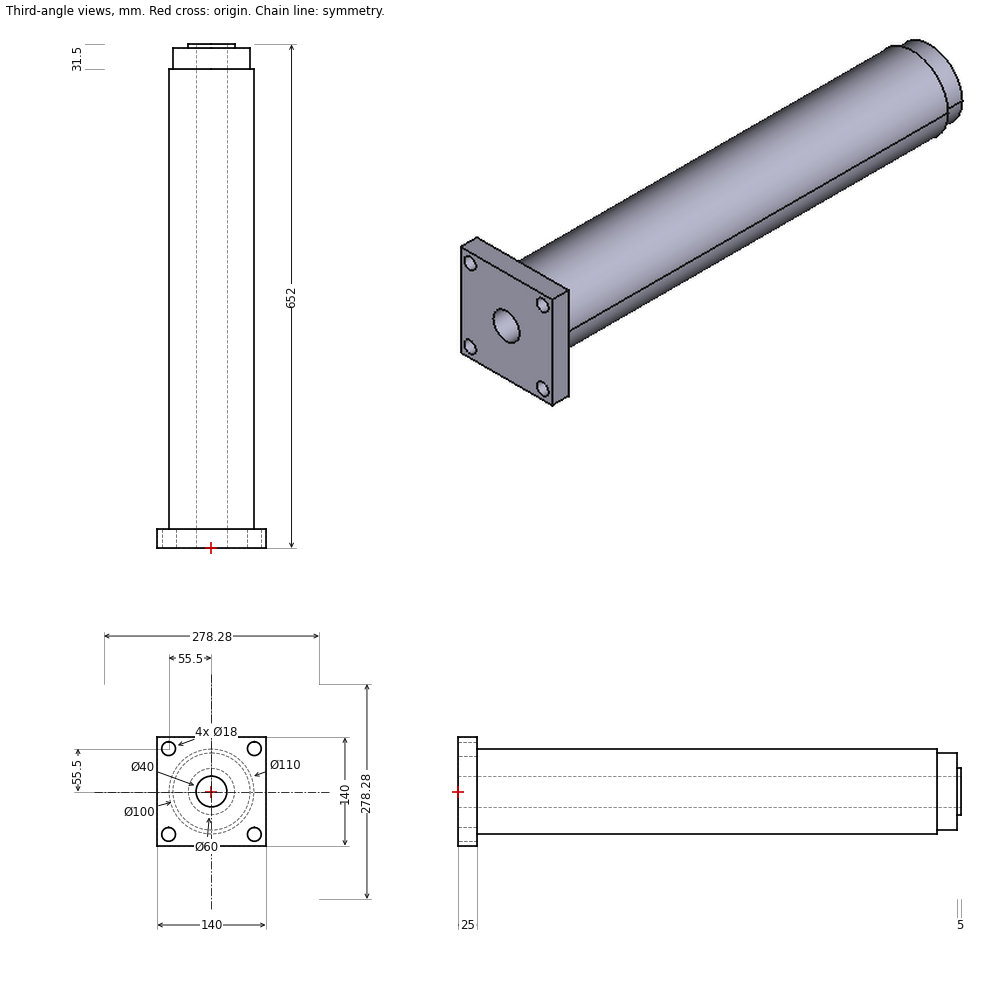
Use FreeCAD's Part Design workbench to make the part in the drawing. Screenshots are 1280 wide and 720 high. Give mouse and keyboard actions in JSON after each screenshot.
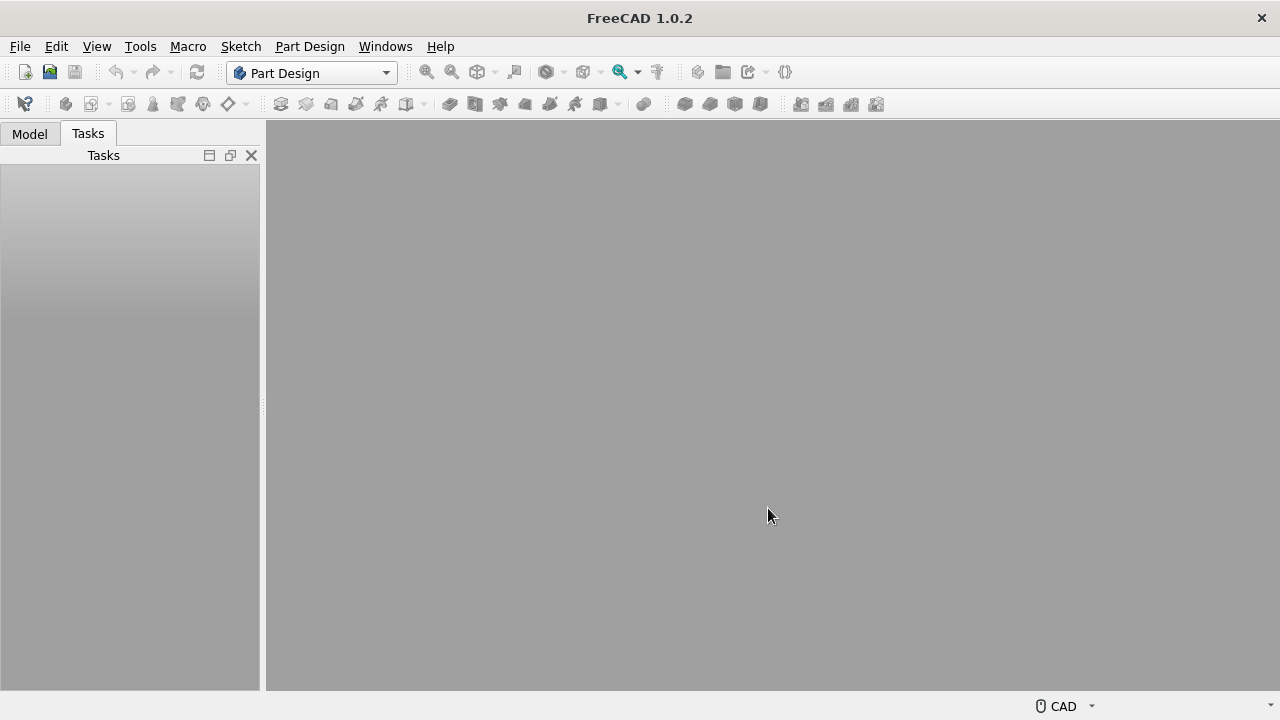
{"action": "left_click", "coordinate": [25, 72]}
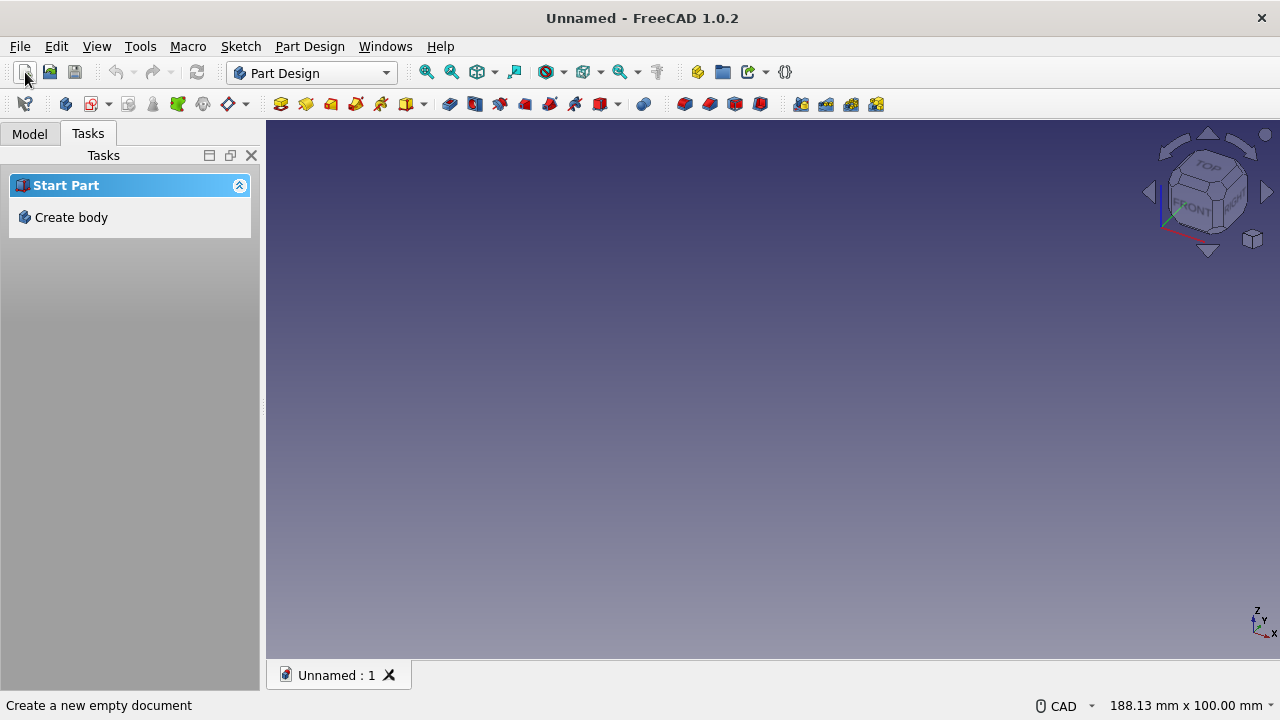
{"action": "left_click", "coordinate": [90, 104]}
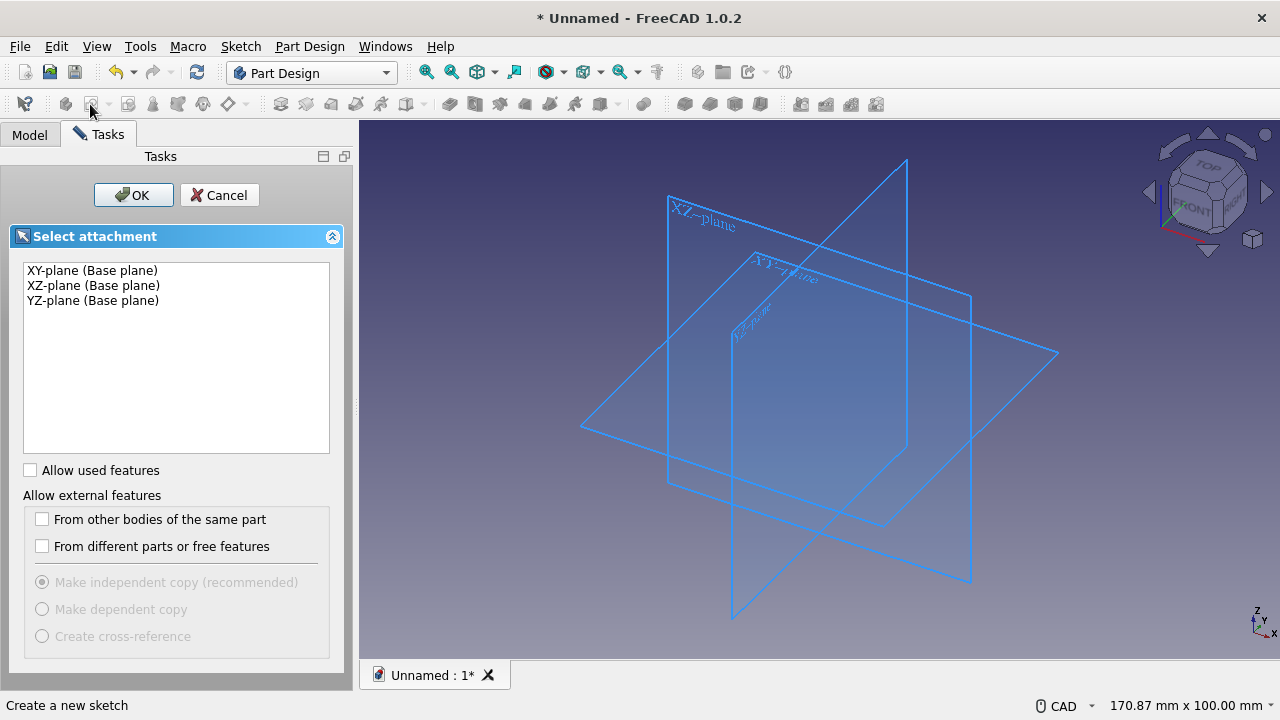
{"action": "left_click", "coordinate": [84, 286]}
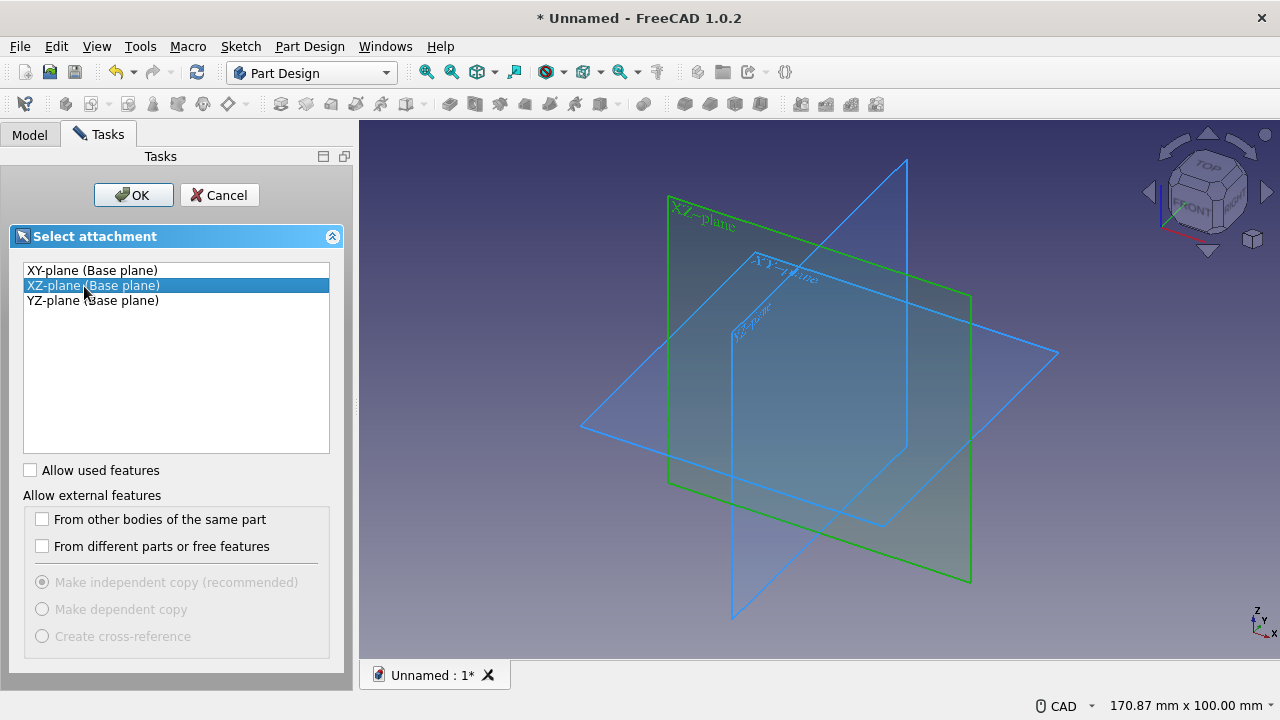
{"action": "left_click", "coordinate": [134, 195]}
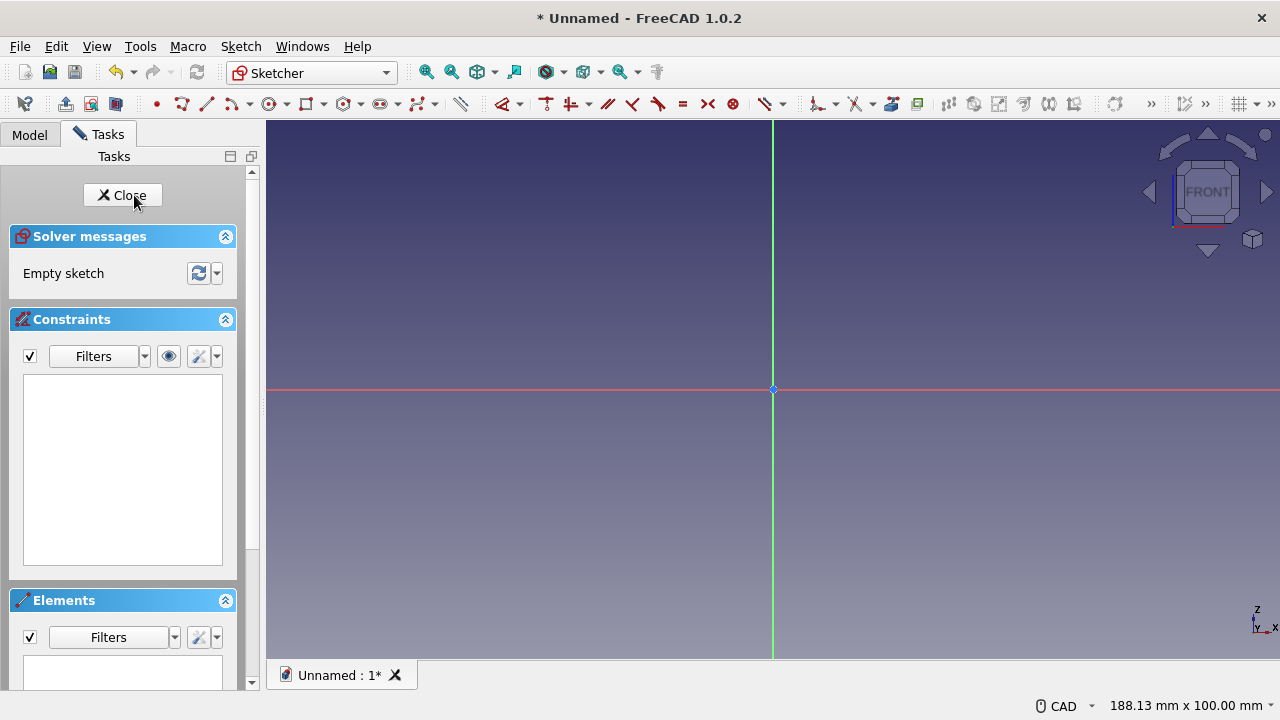
{"action": "scroll", "coordinate": [649, 390], "scroll_direction": "down", "scroll_amount": 4}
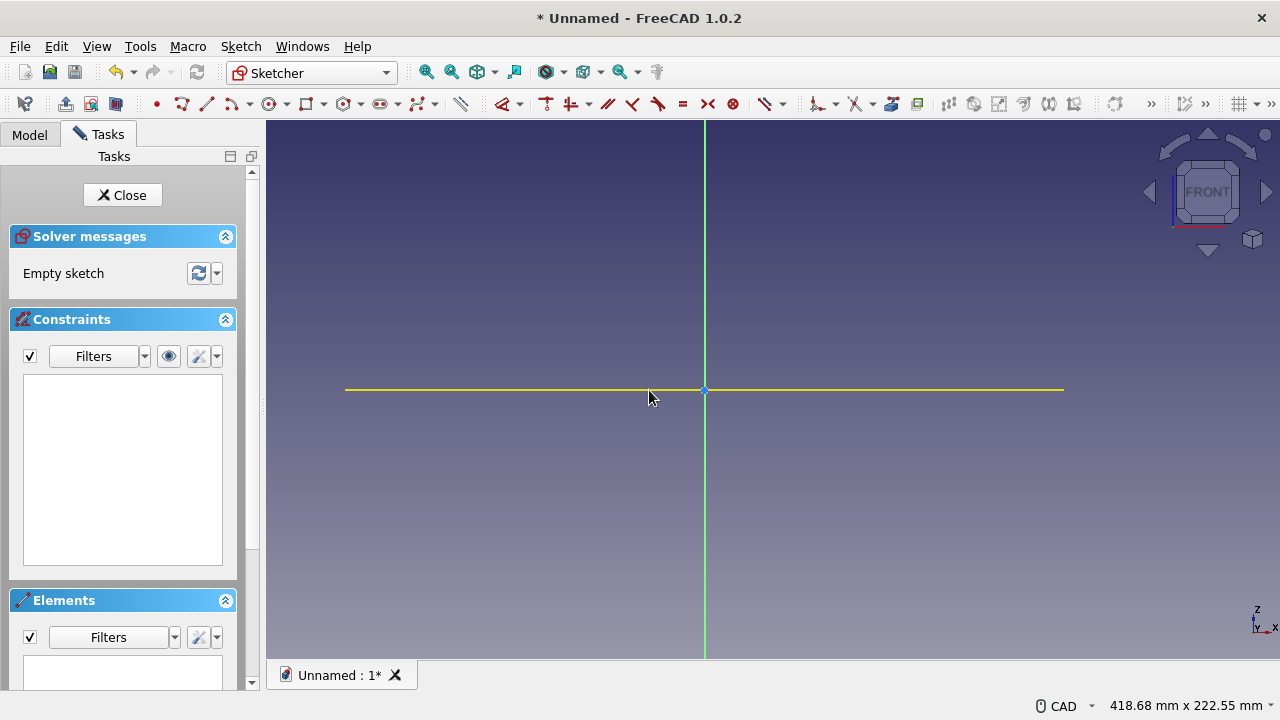
{"action": "left_click", "coordinate": [324, 104]}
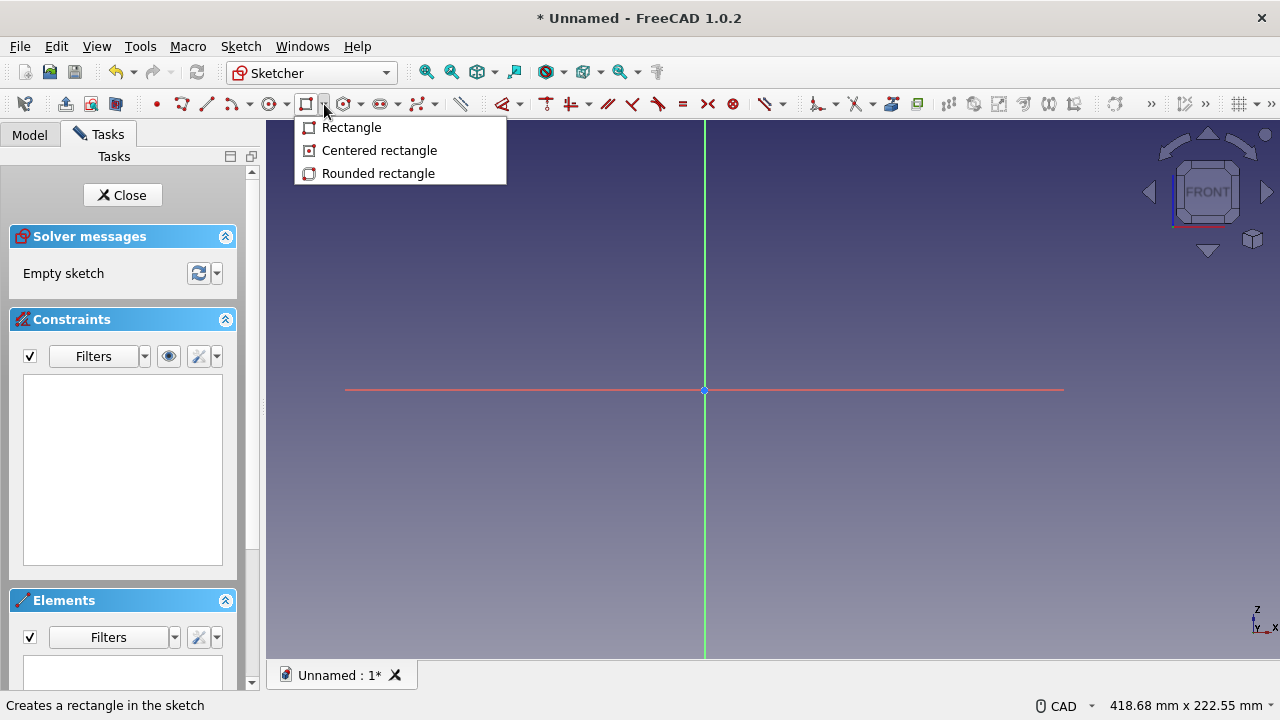
{"action": "left_click", "coordinate": [400, 150]}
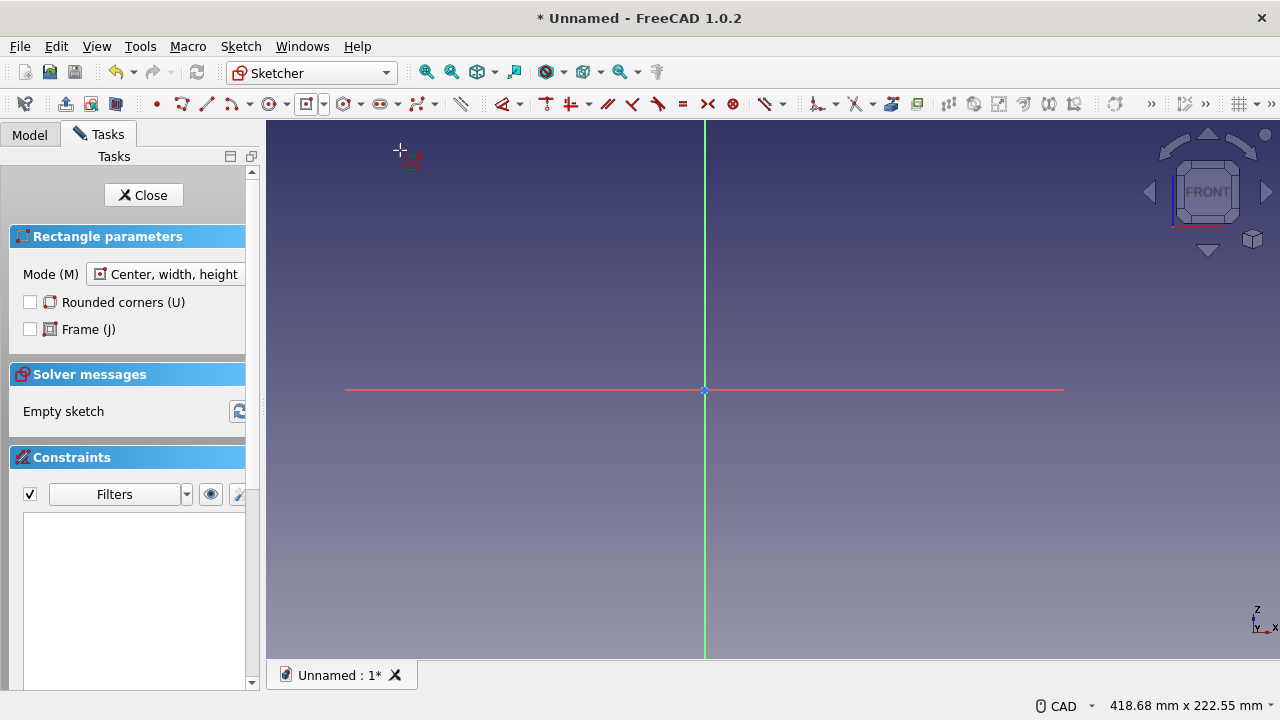
{"action": "left_click", "coordinate": [705, 390]}
{"action": "mouse_move", "coordinate": [874, 221]}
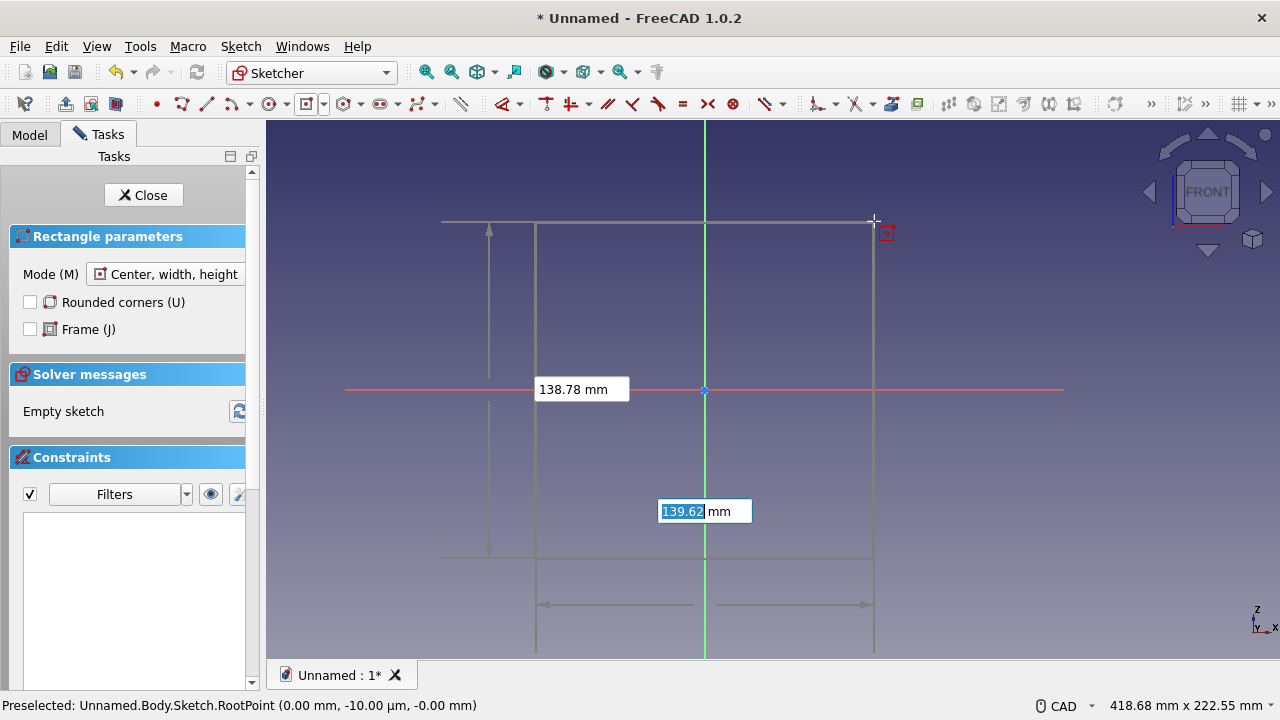
{"action": "type", "text": "140"}
{"action": "key", "text": "Tab"}
{"action": "type", "text": "140"}
{"action": "key", "text": "Return"}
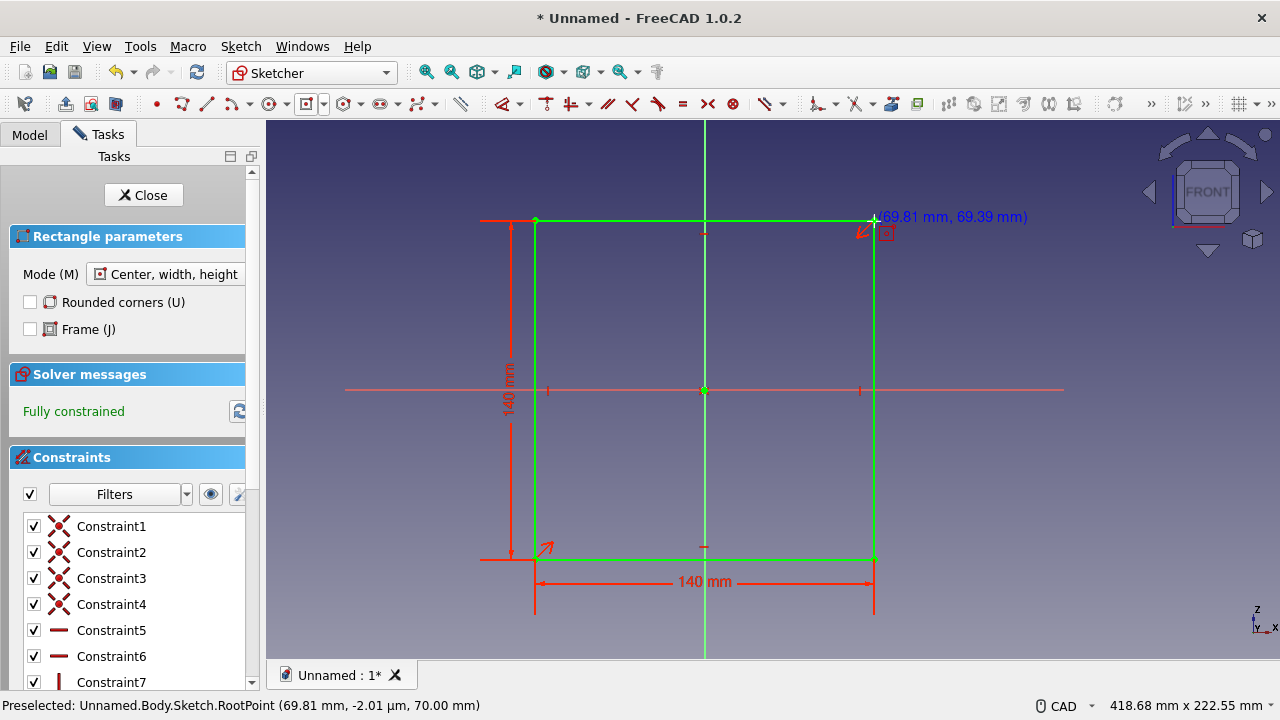
{"action": "left_click", "coordinate": [268, 104]}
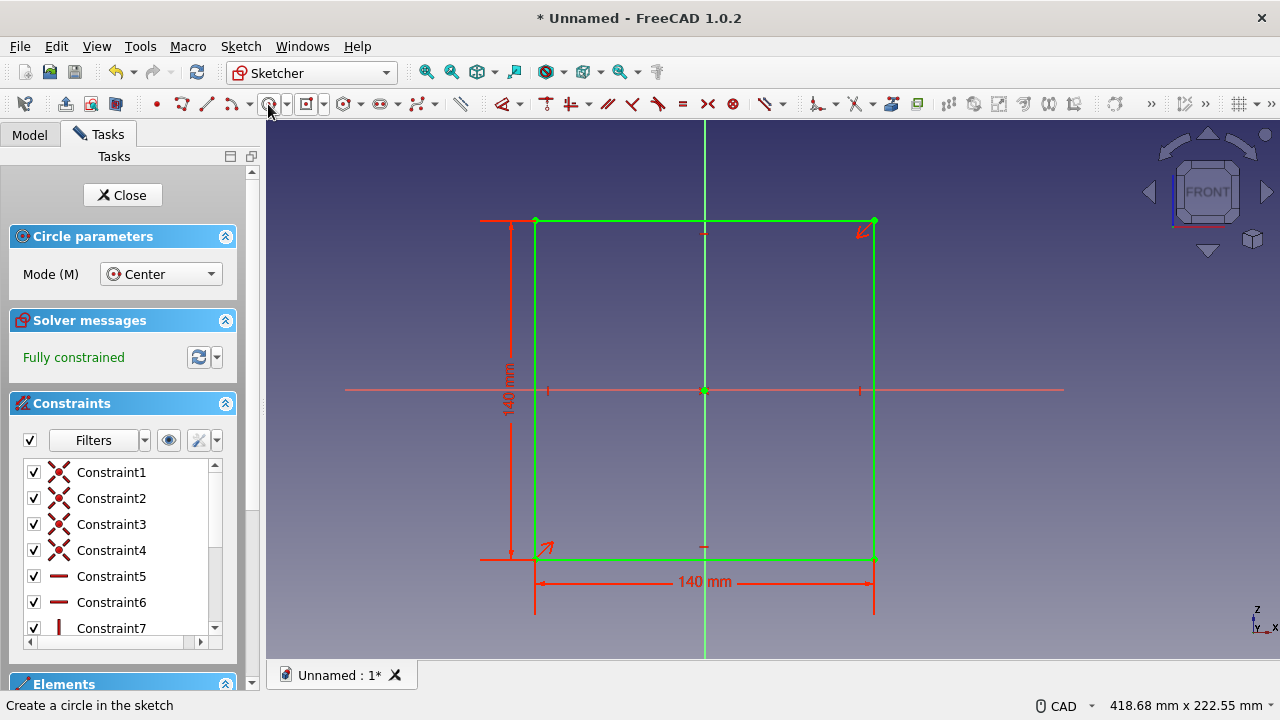
{"action": "left_click", "coordinate": [571, 256]}
{"action": "mouse_move", "coordinate": [586, 240]}